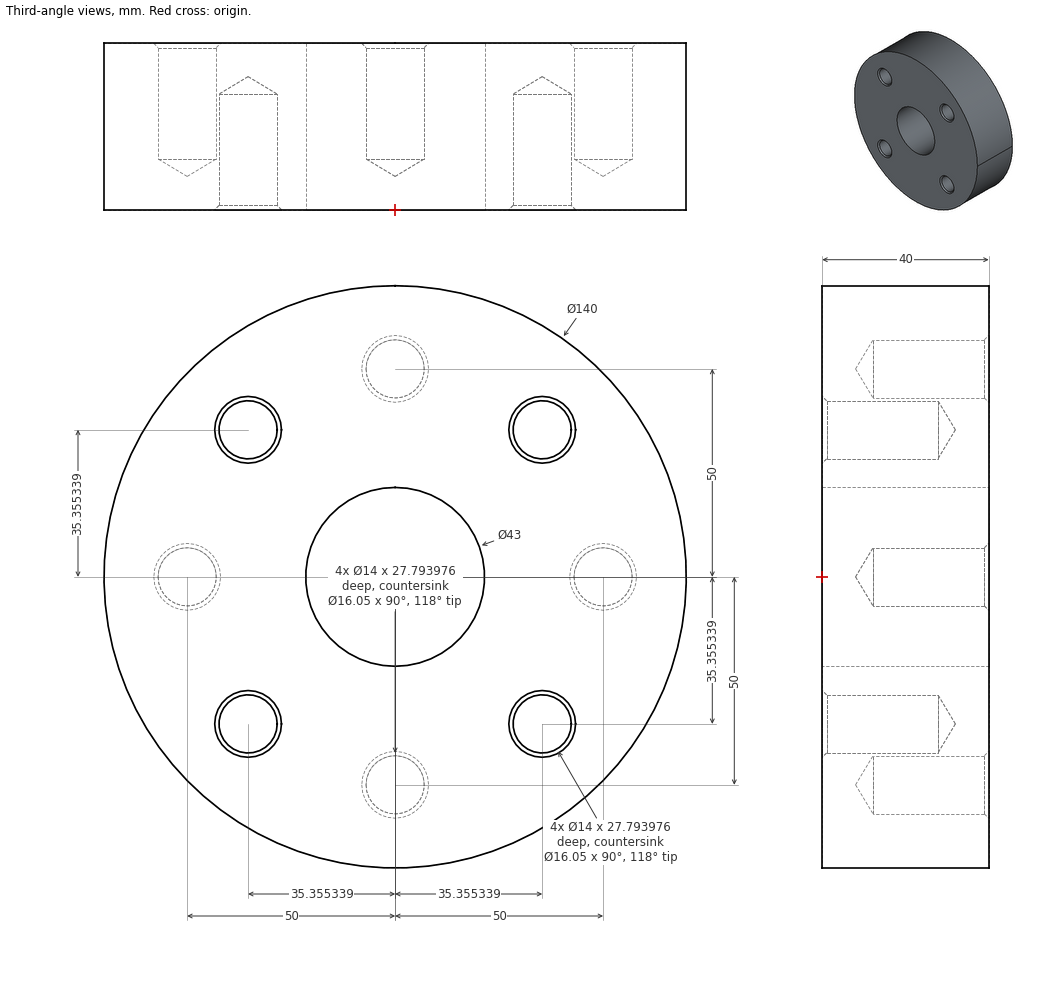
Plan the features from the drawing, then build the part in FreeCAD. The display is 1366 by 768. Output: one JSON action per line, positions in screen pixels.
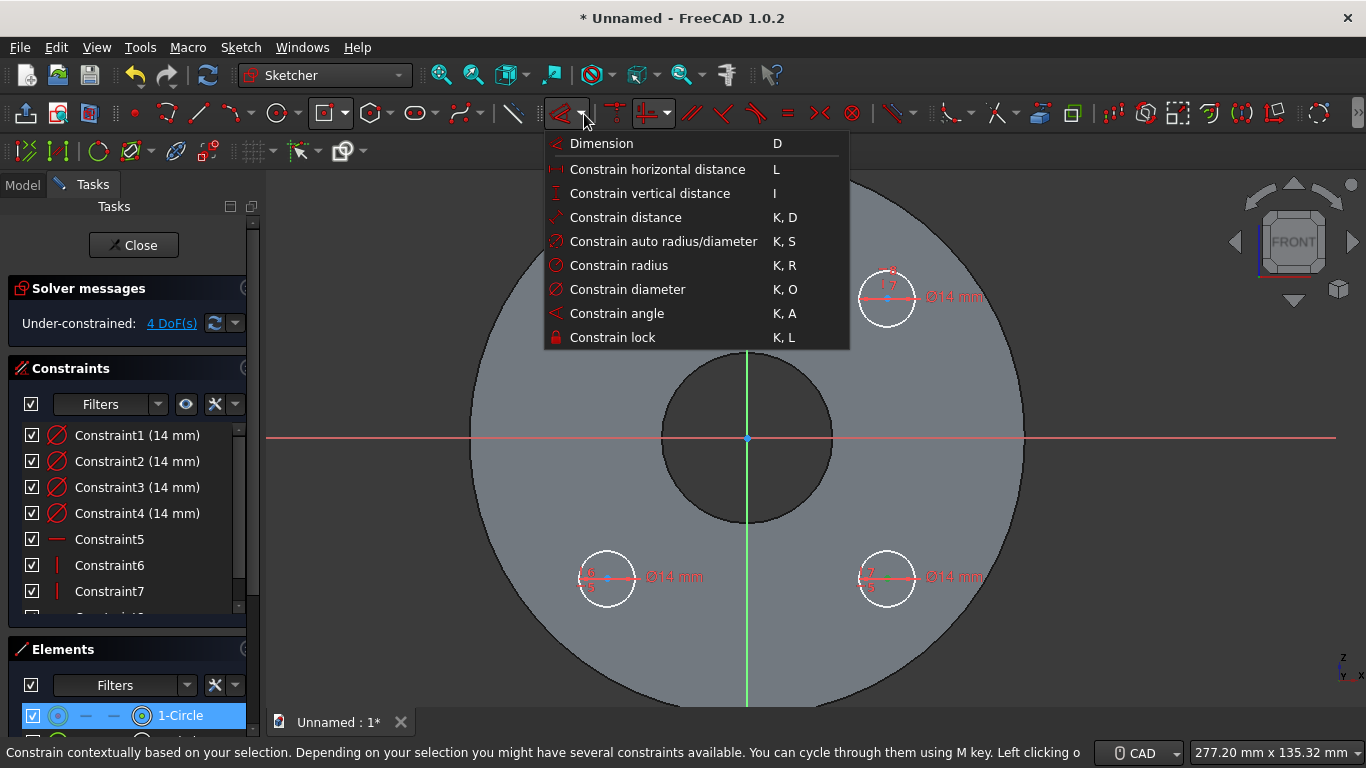
{"action": "left_click", "coordinate": [697, 169]}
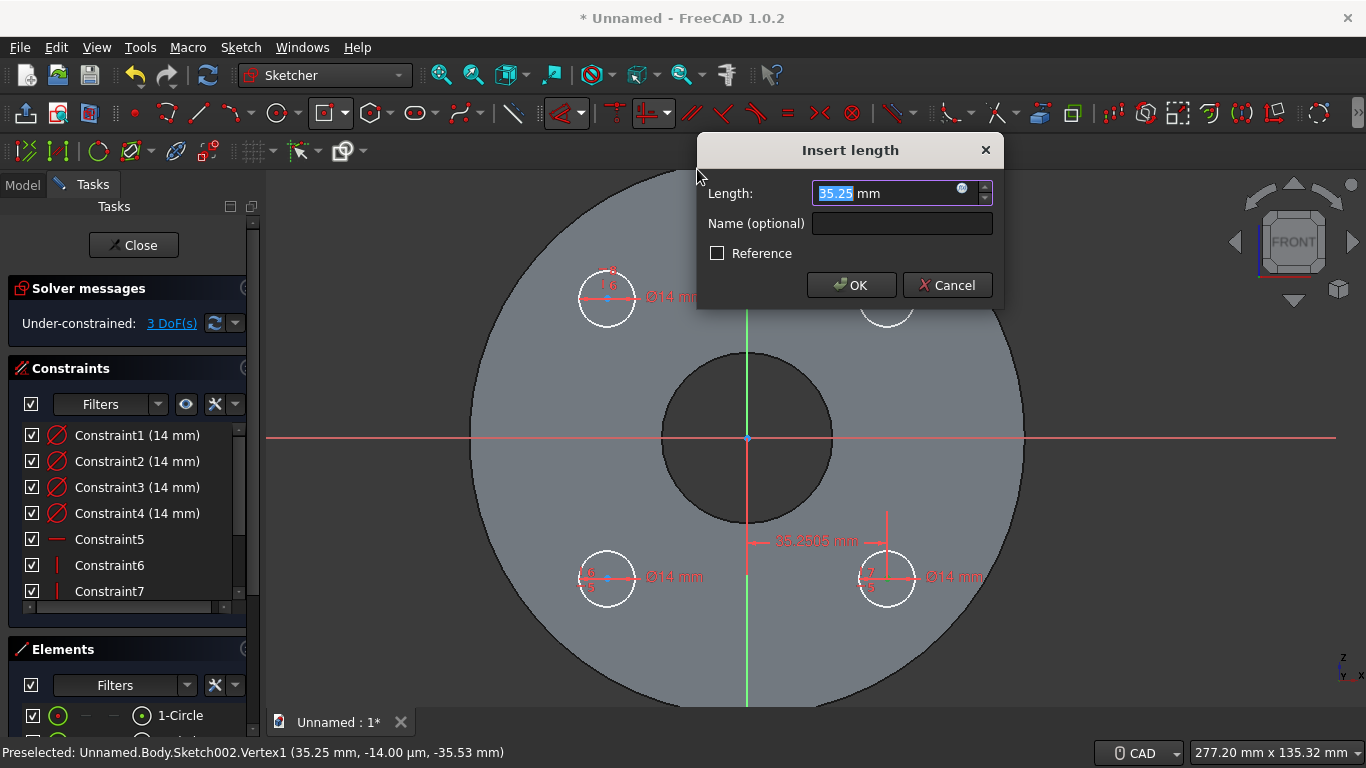
{"action": "type", "text": "35.355339"}
{"action": "key", "text": "Return"}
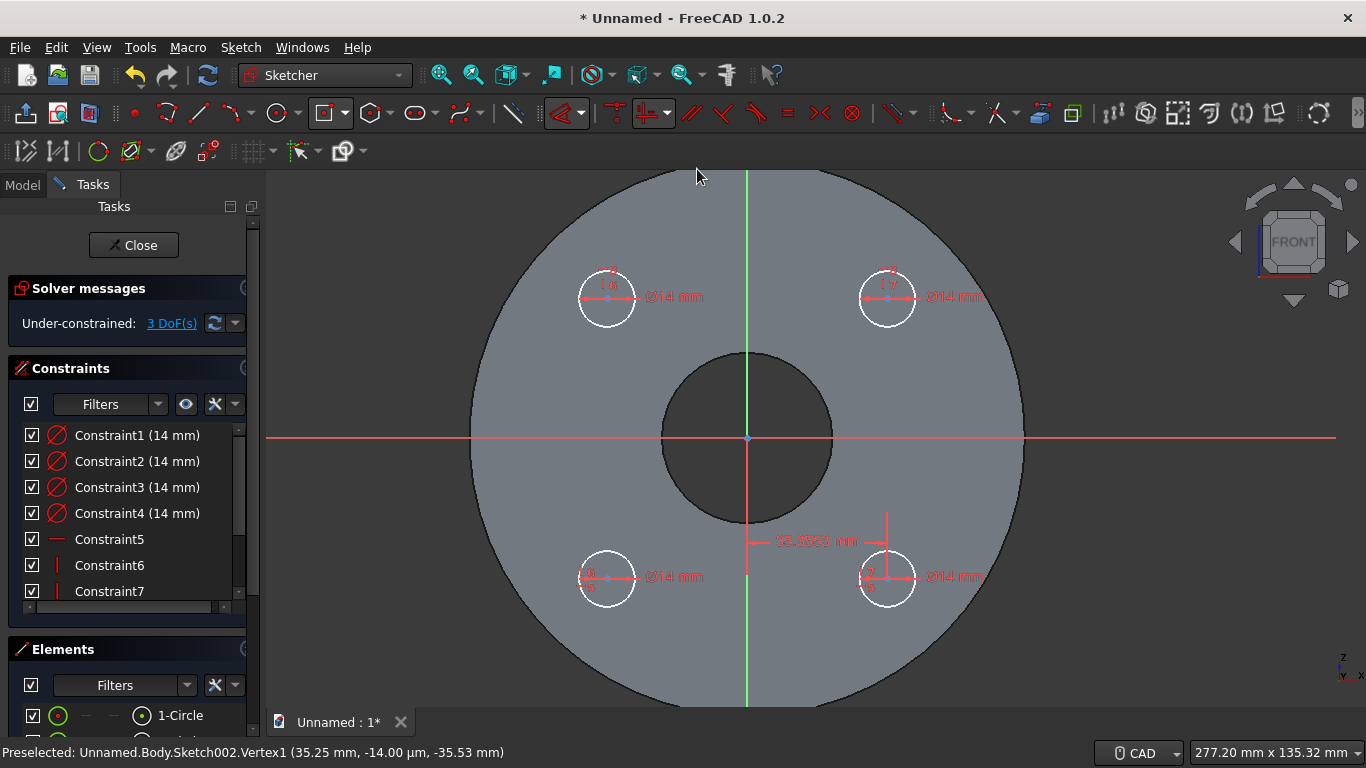
{"action": "left_click", "coordinate": [887, 579]}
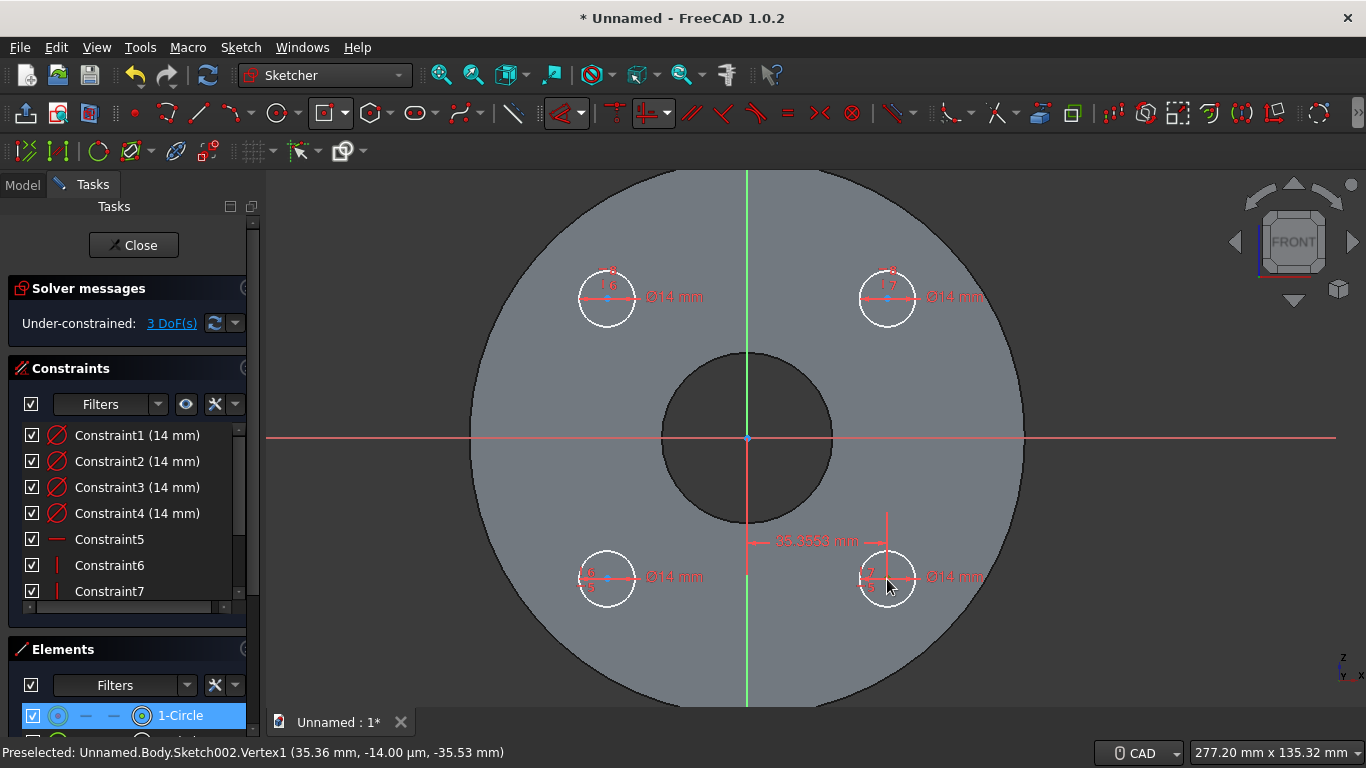
{"action": "key", "text": "i"}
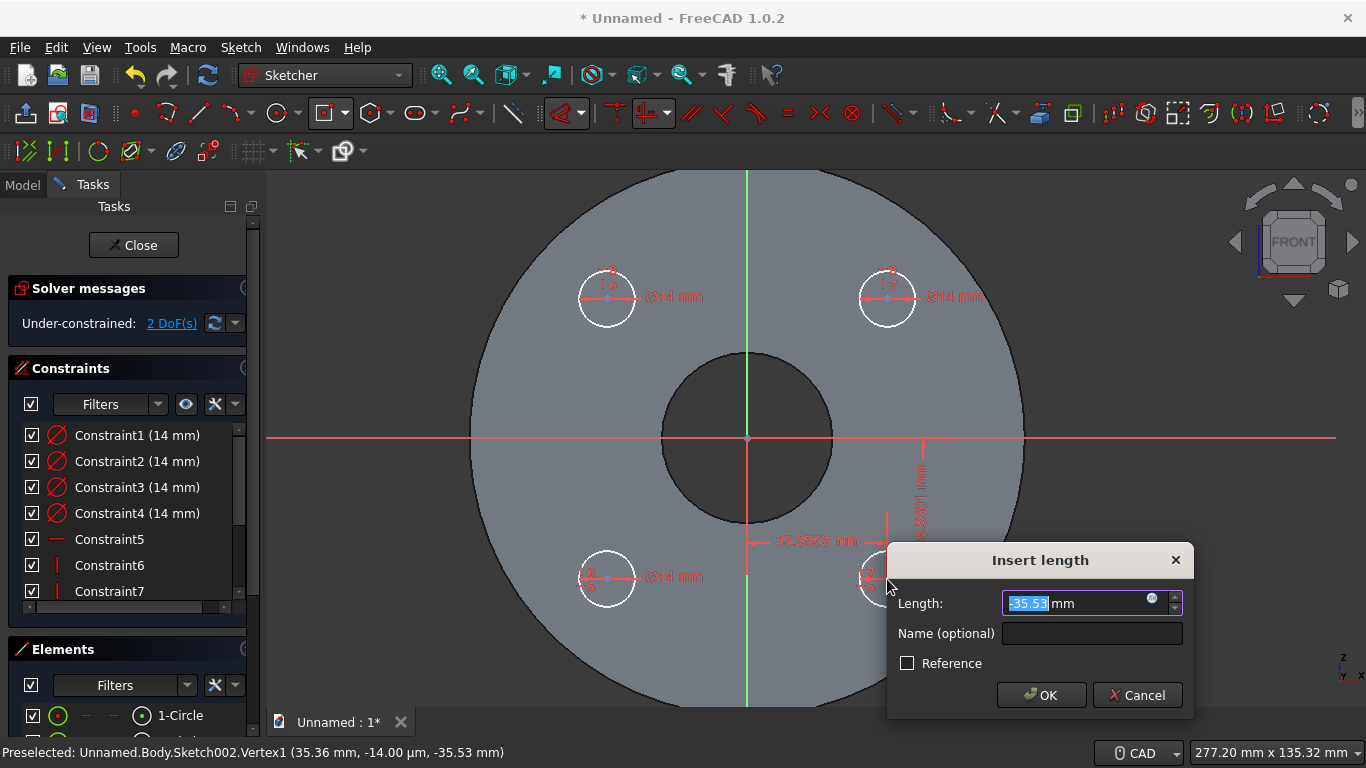
{"action": "type", "text": "-35.355339"}
{"action": "key", "text": "Return"}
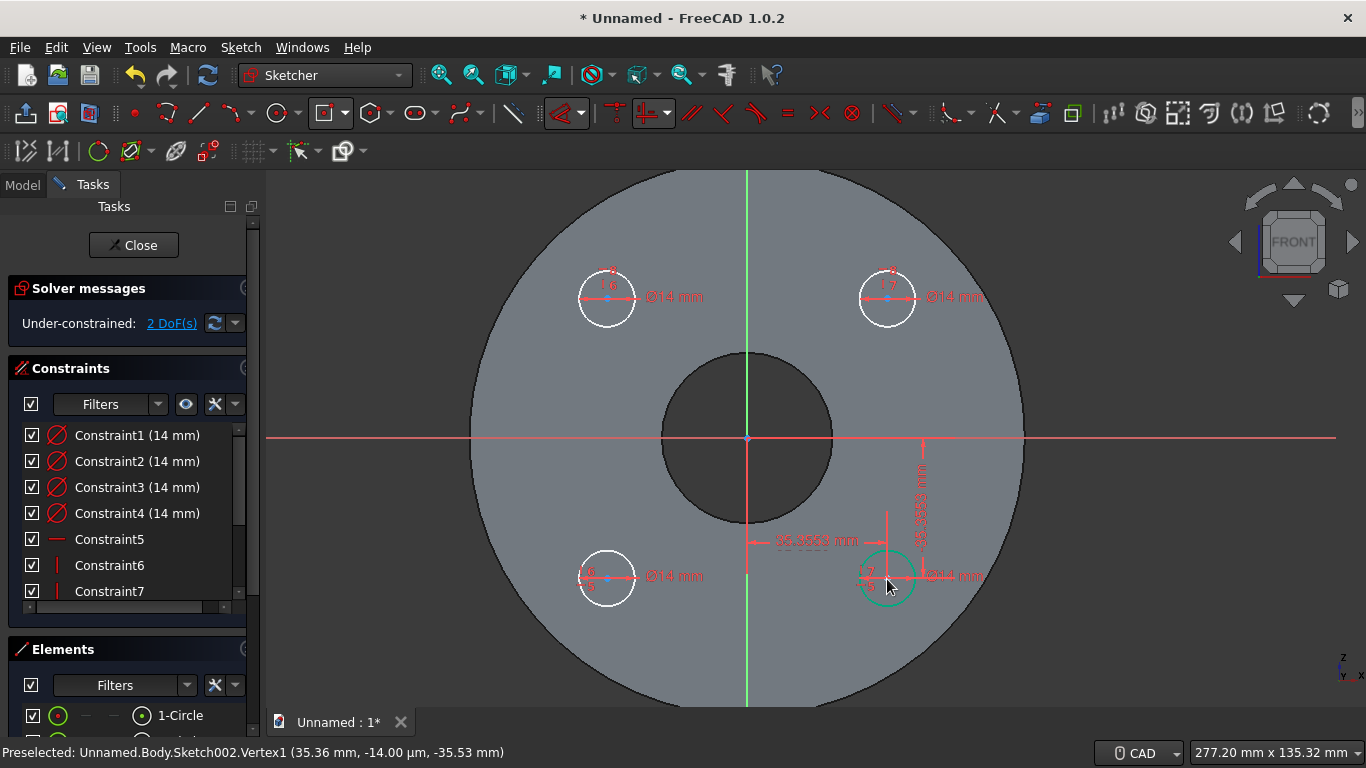
{"action": "left_click", "coordinate": [607, 578]}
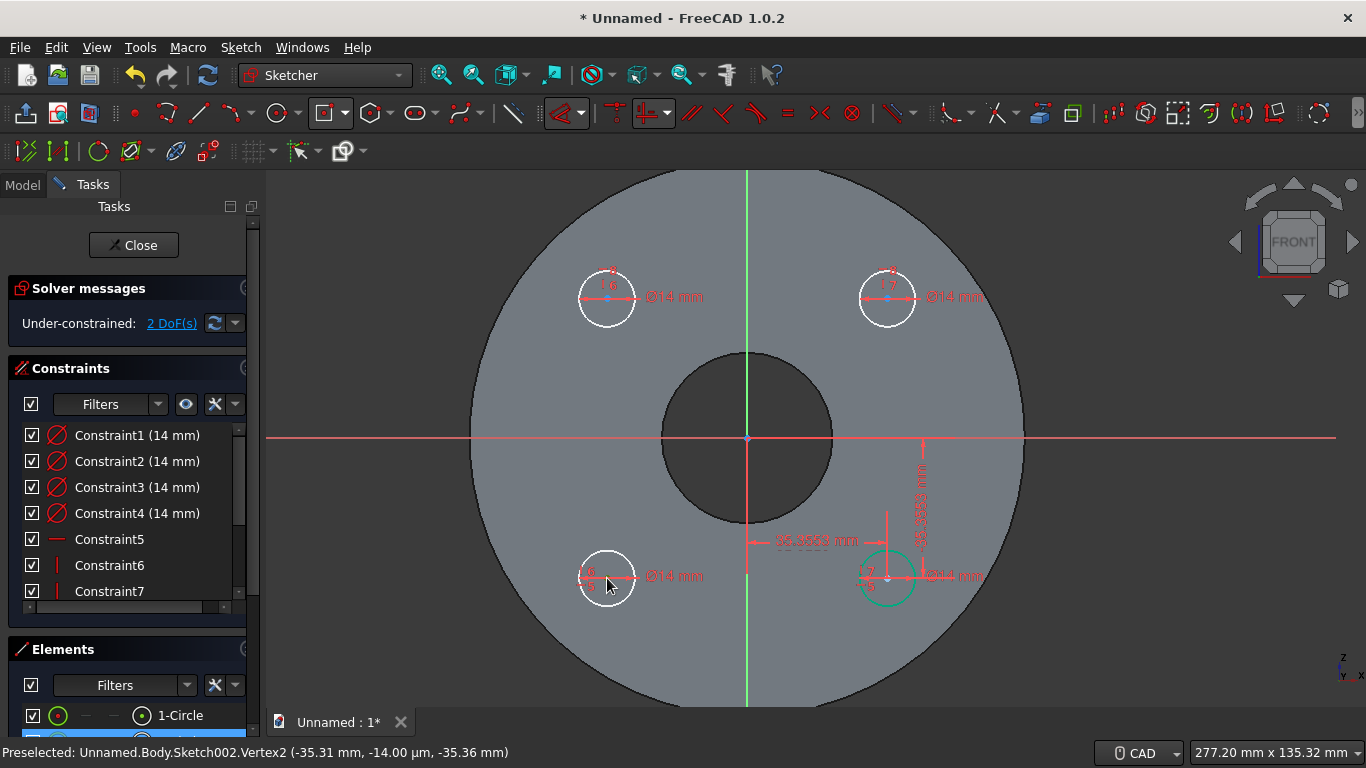
{"action": "left_click", "coordinate": [584, 114]}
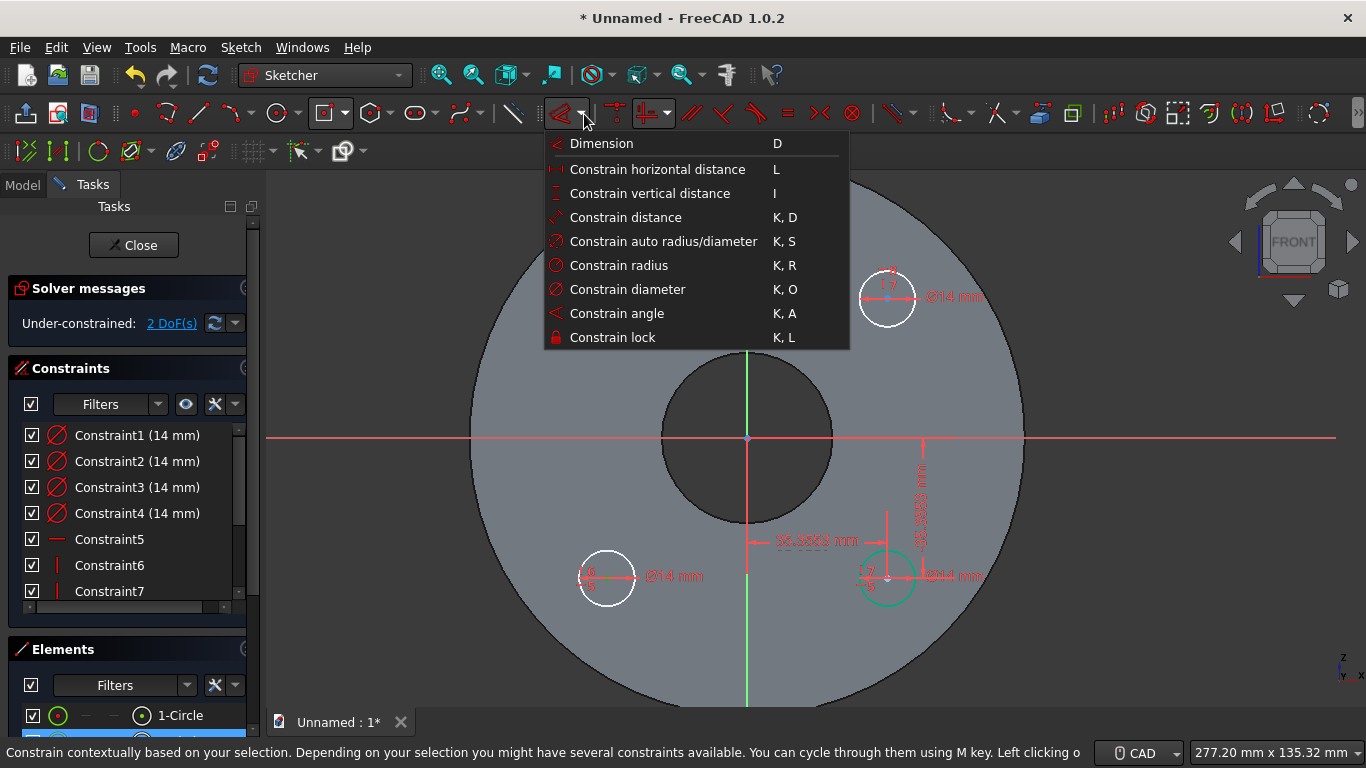
{"action": "left_click", "coordinate": [697, 169]}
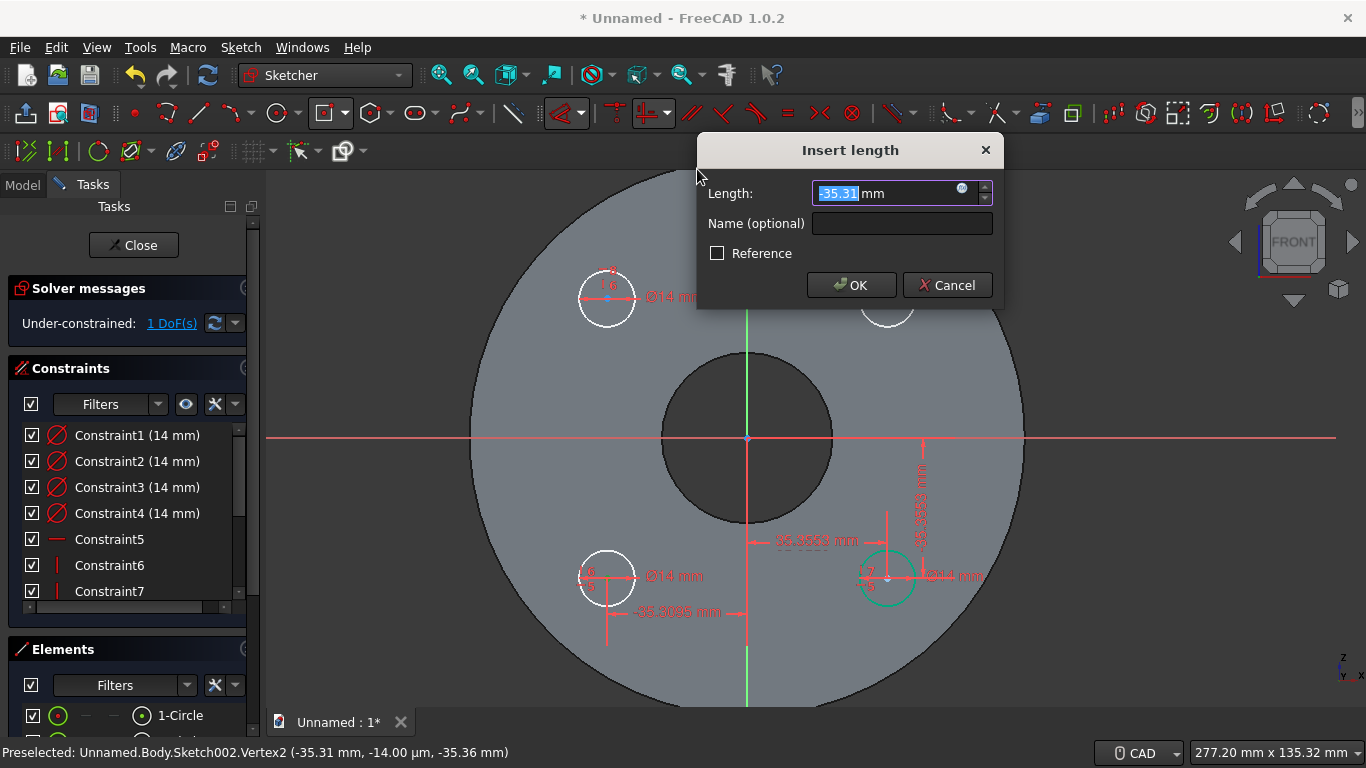
{"action": "type", "text": "-35.355339"}
{"action": "key", "text": "Return"}